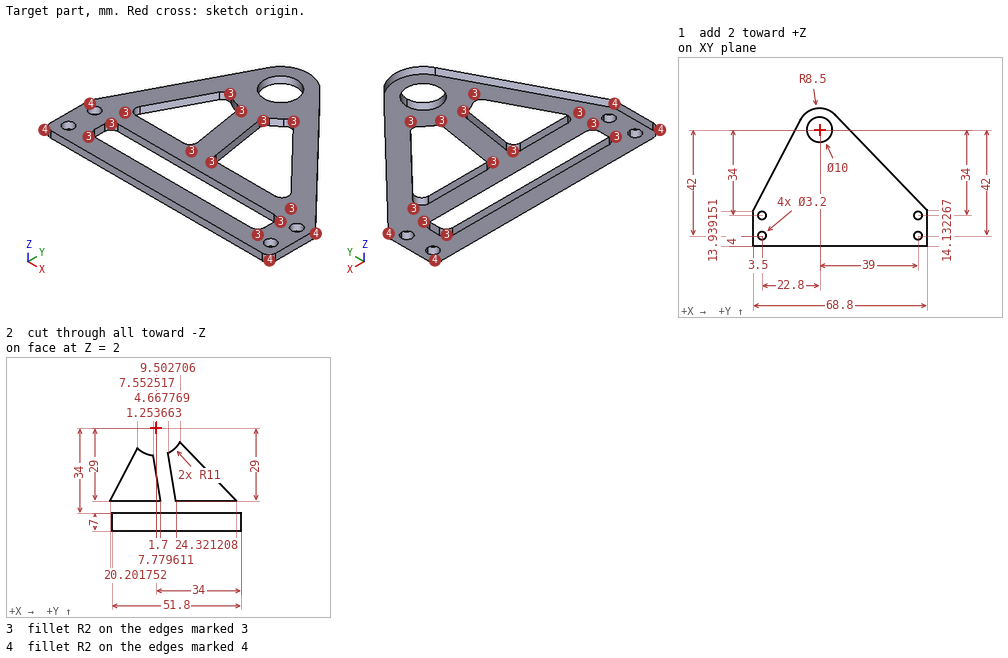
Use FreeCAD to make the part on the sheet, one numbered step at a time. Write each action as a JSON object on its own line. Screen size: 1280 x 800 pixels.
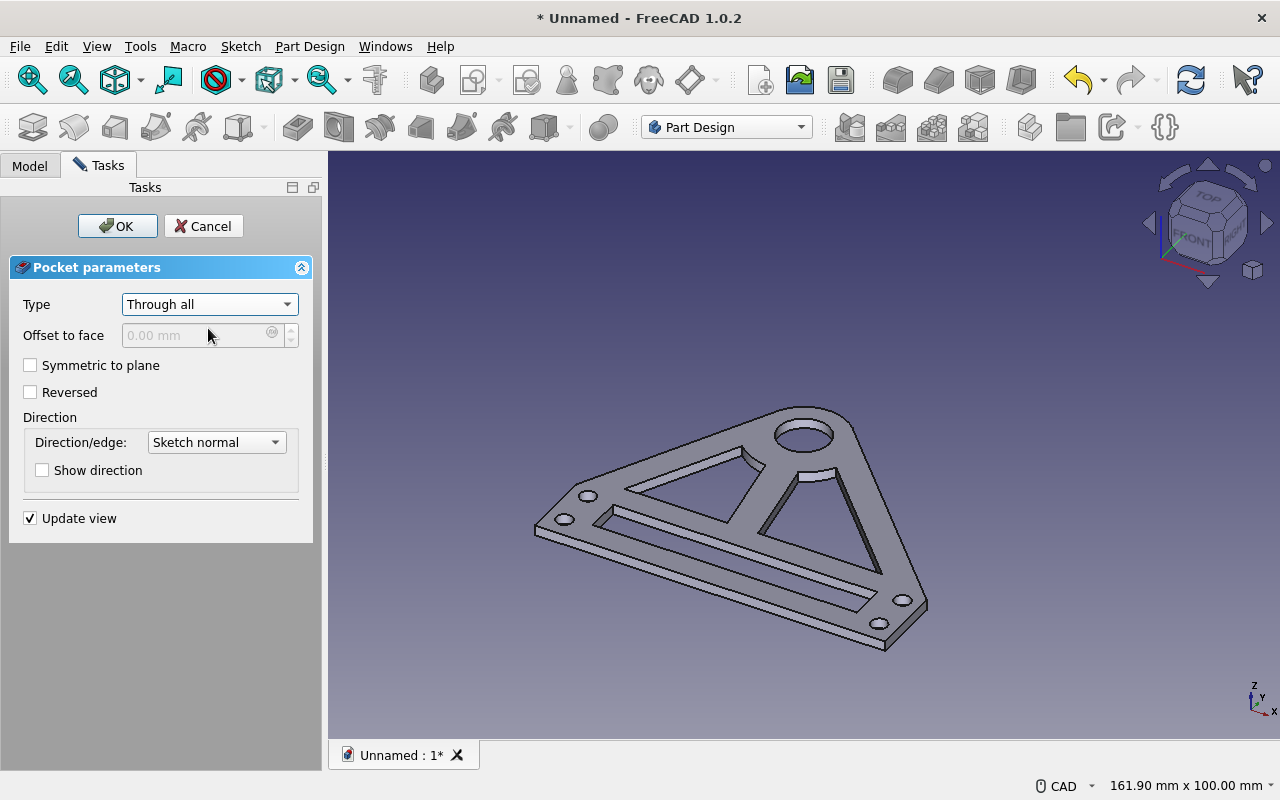
{"action": "left_click", "coordinate": [118, 226]}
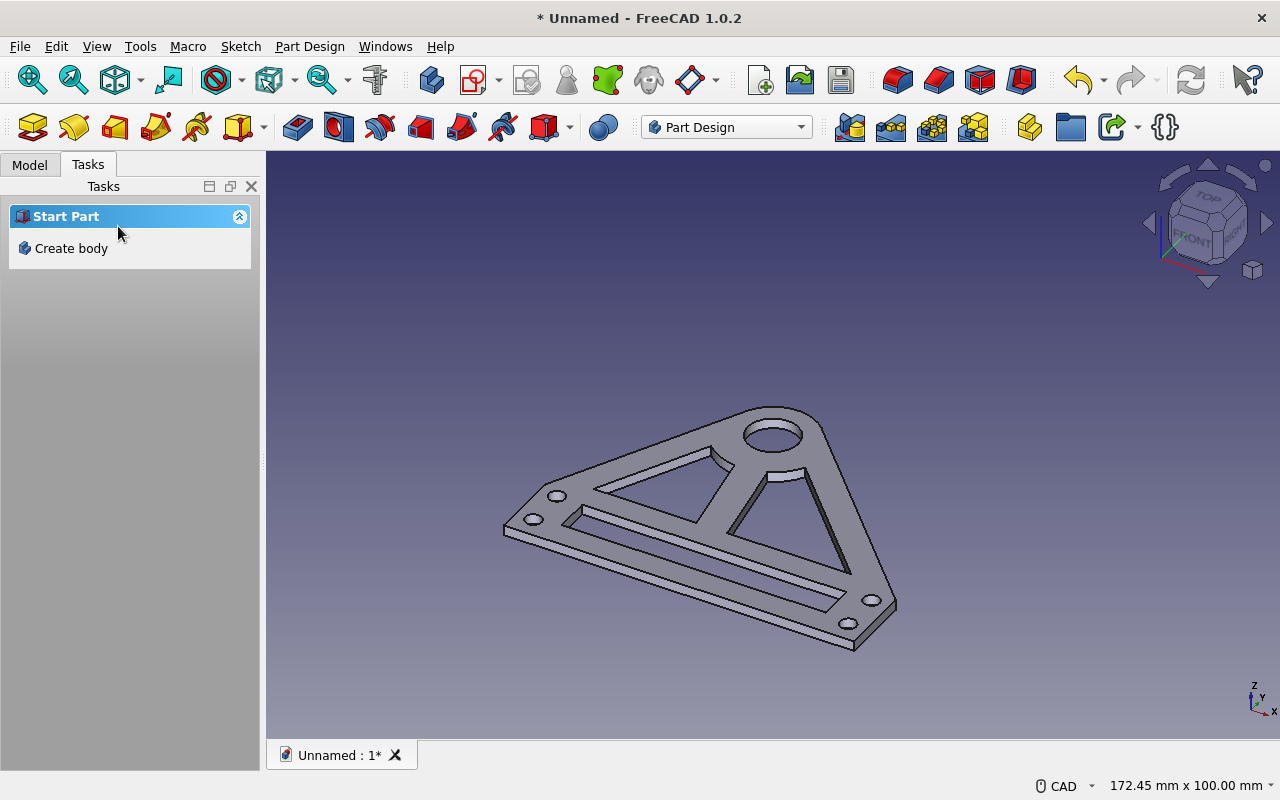
{"action": "scroll", "coordinate": [562, 529], "scroll_direction": "up", "scroll_amount": 7}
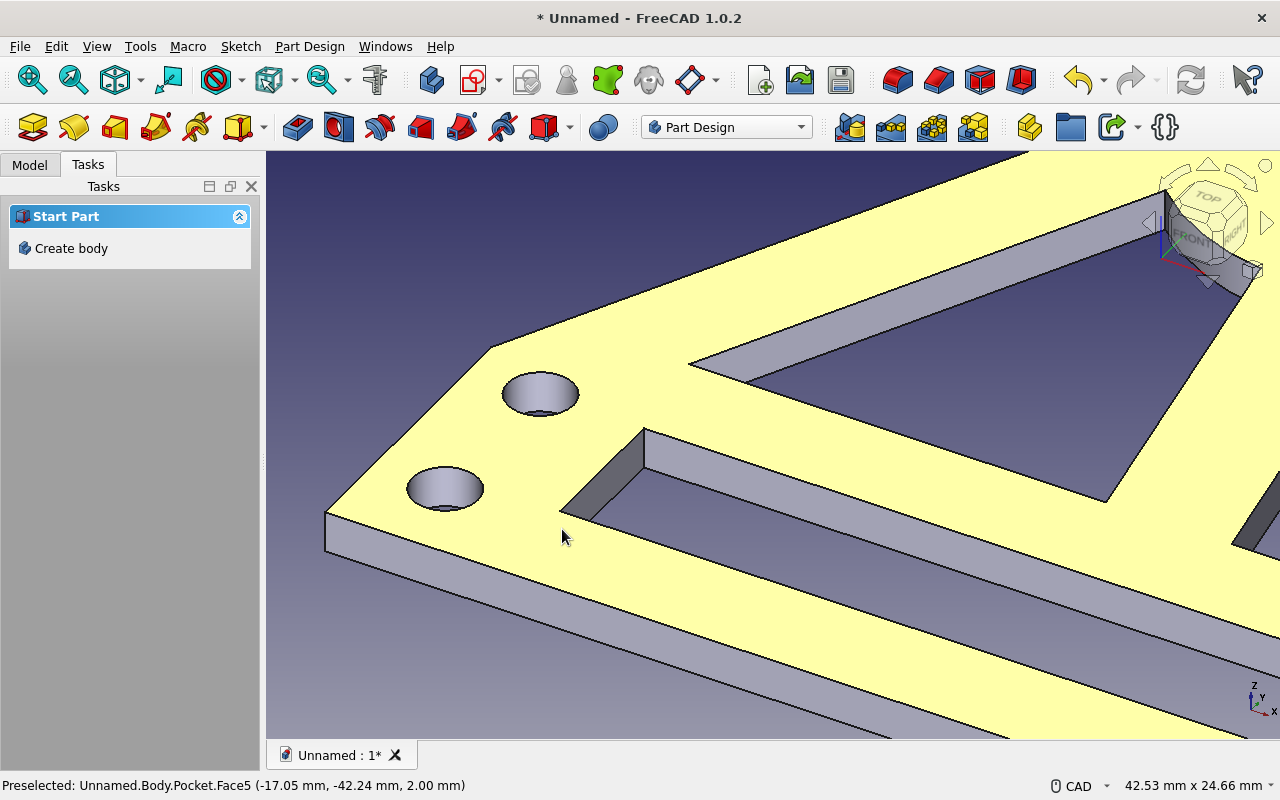
{"action": "left_click", "coordinate": [33, 80]}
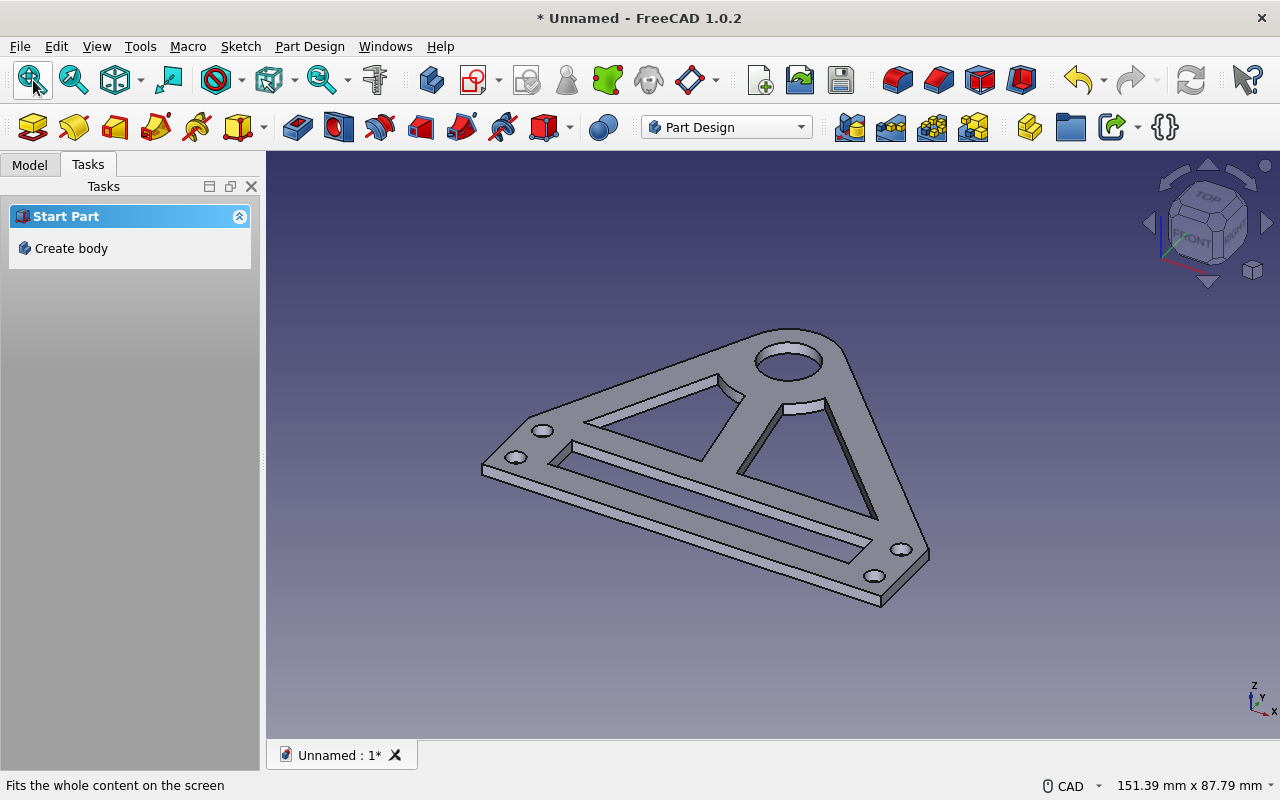
{"action": "key", "text": "0"}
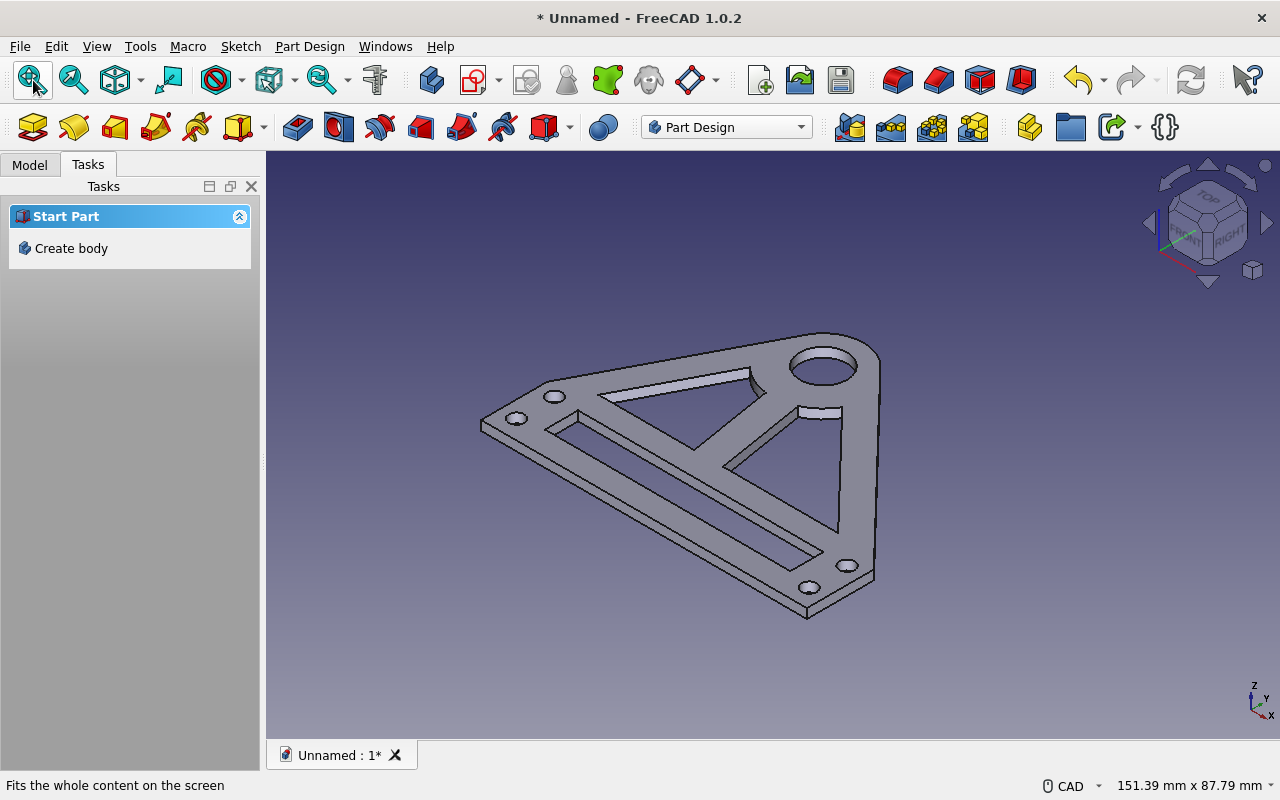
{"action": "scroll", "coordinate": [545, 434], "scroll_direction": "up", "scroll_amount": 6}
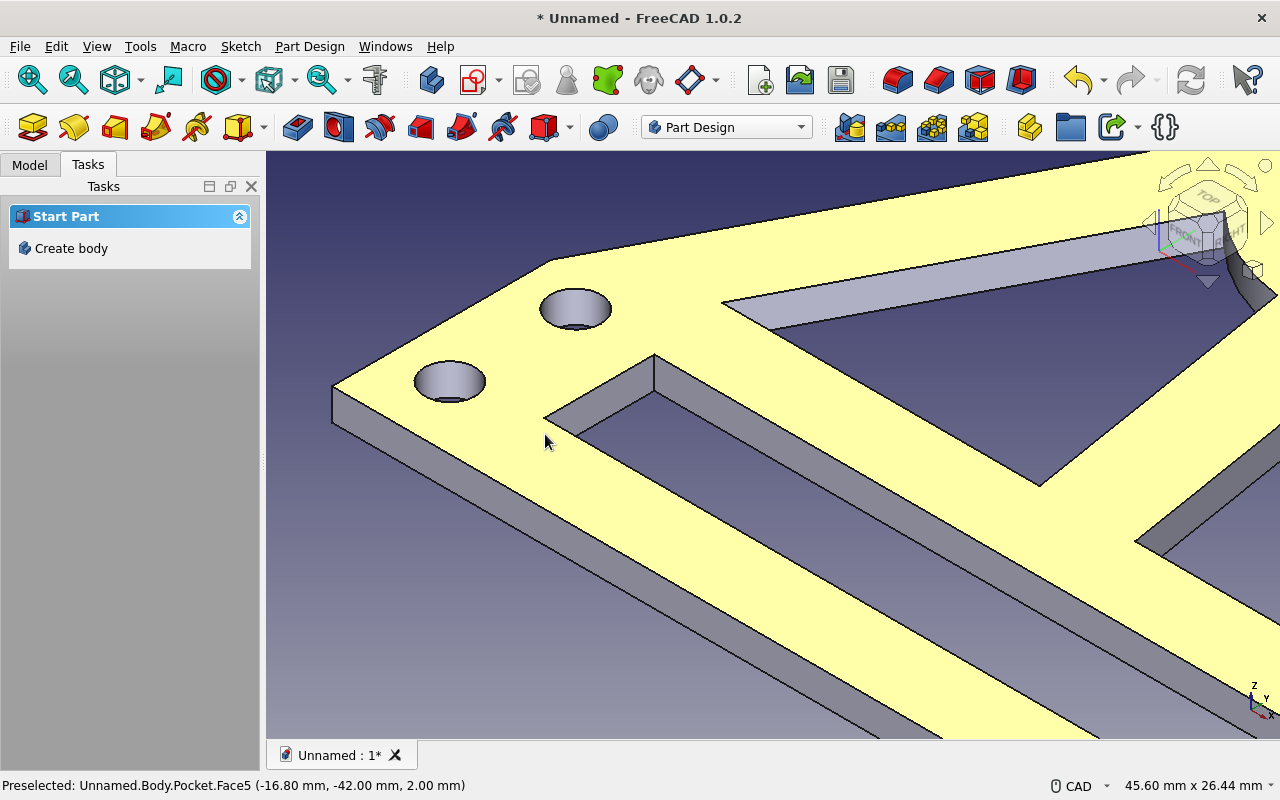
{"action": "key", "text": "v f"}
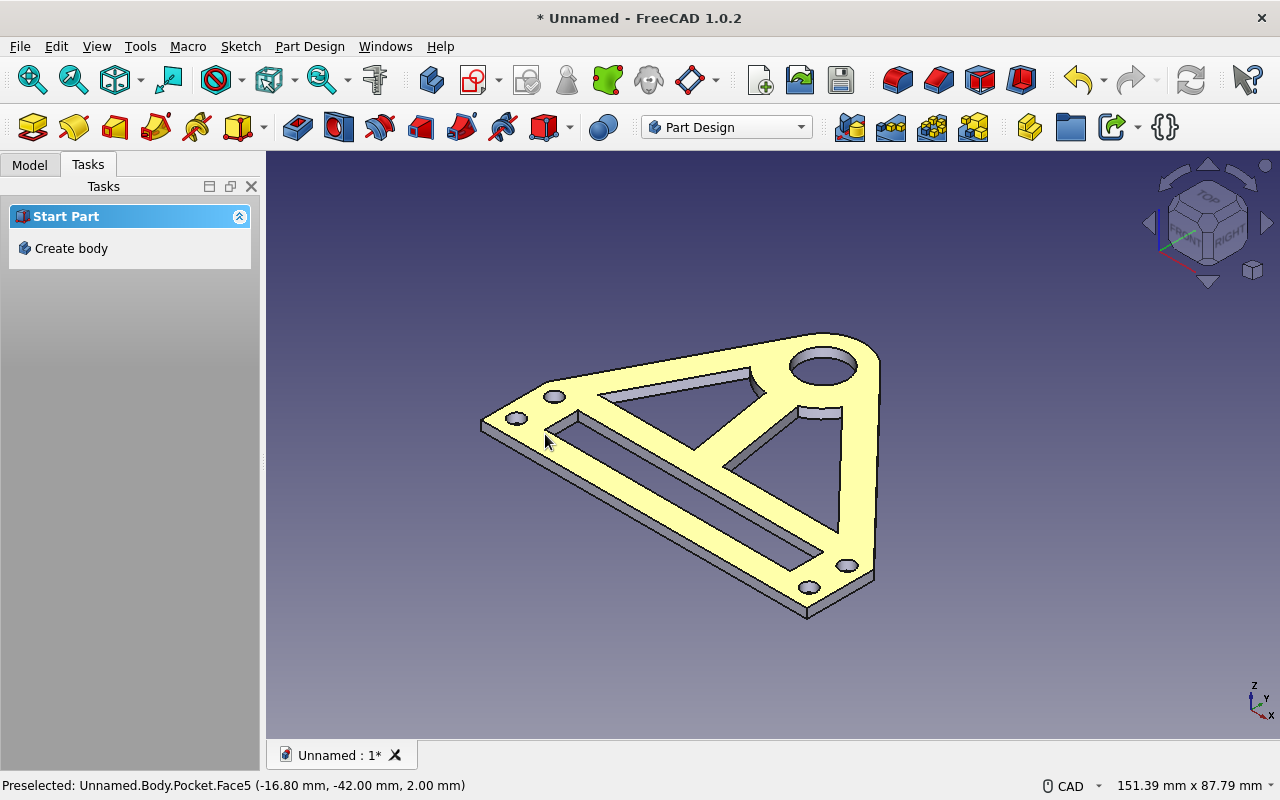
{"action": "key", "text": "2"}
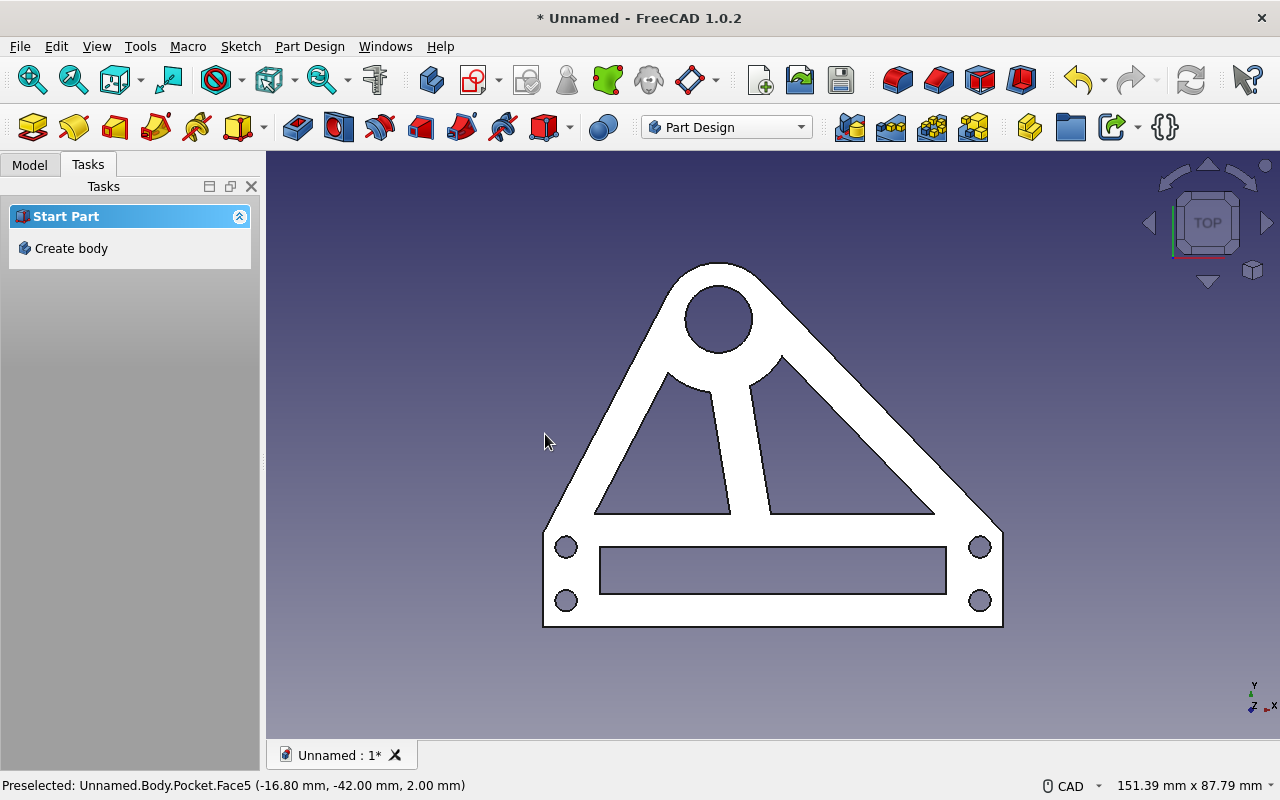
{"action": "scroll", "coordinate": [600, 593], "scroll_direction": "up", "scroll_amount": 6}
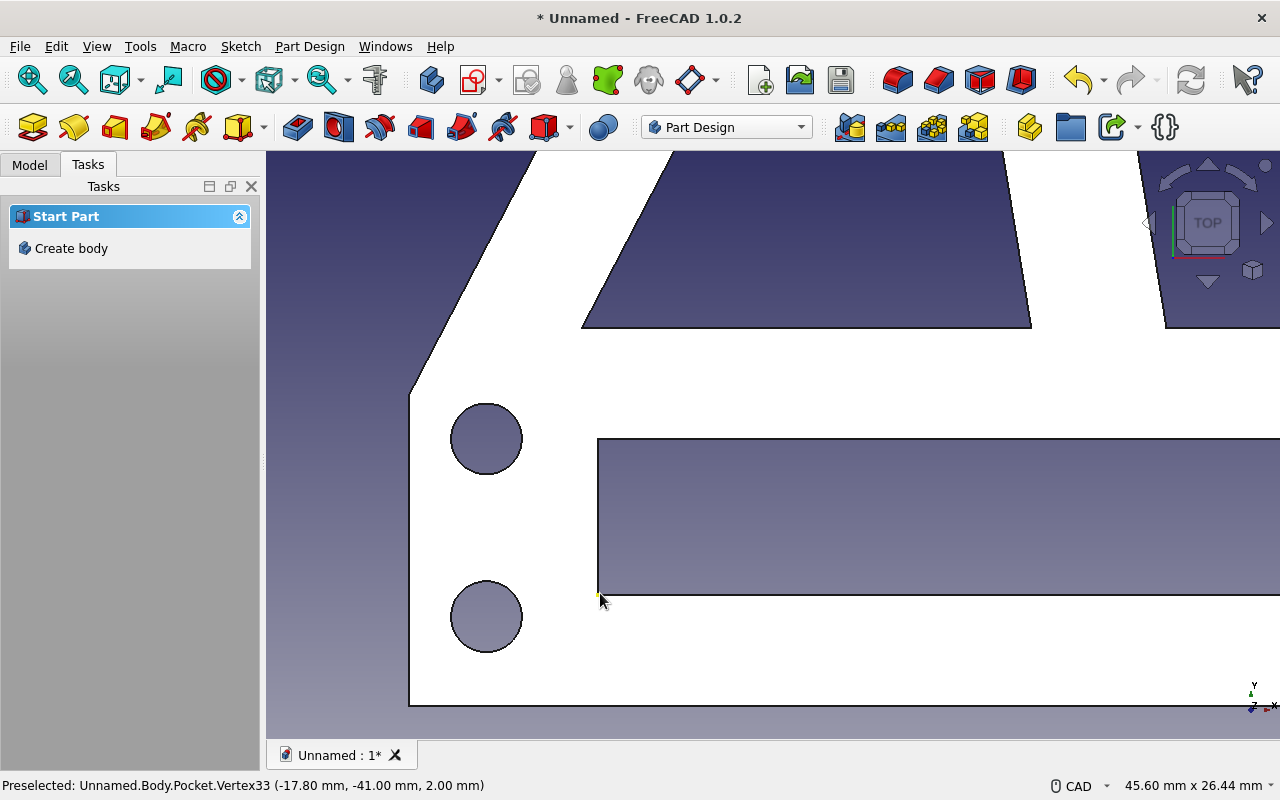
{"action": "left_click", "coordinate": [33, 80]}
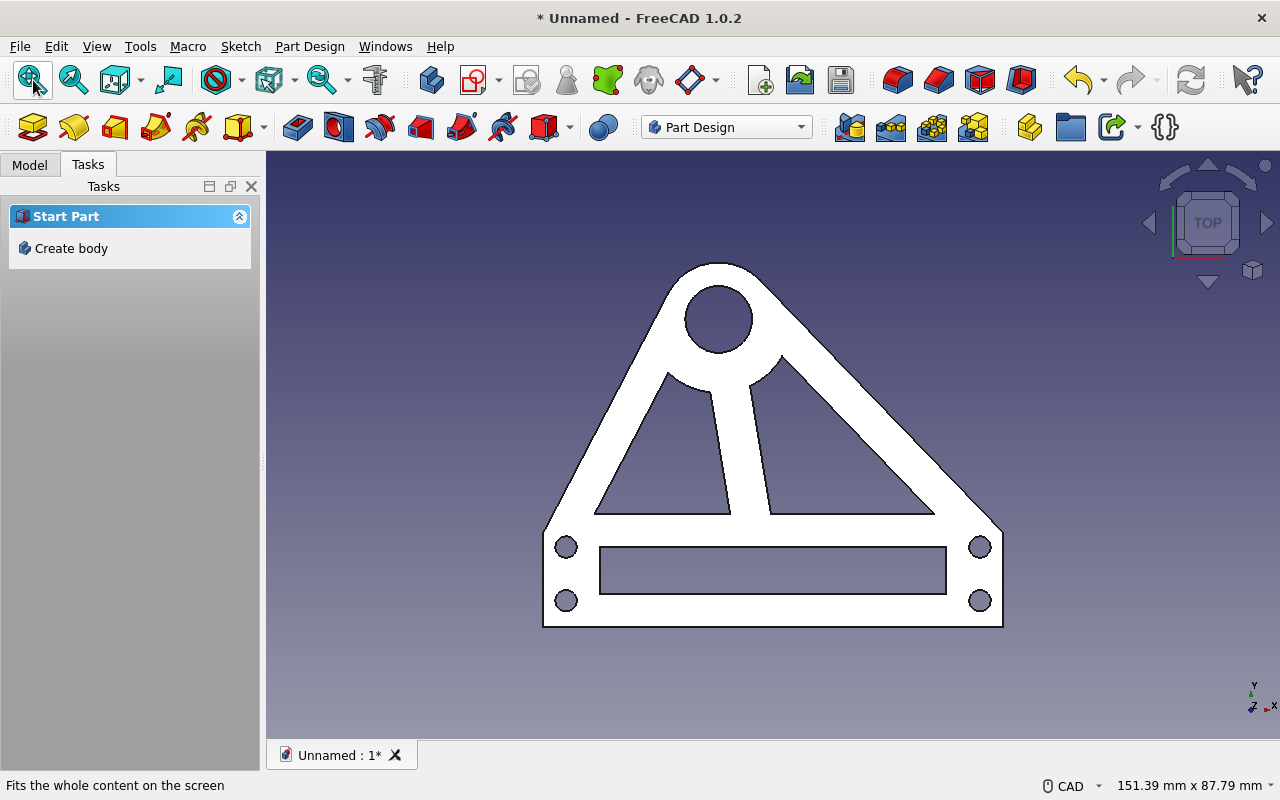
{"action": "key", "text": "1"}